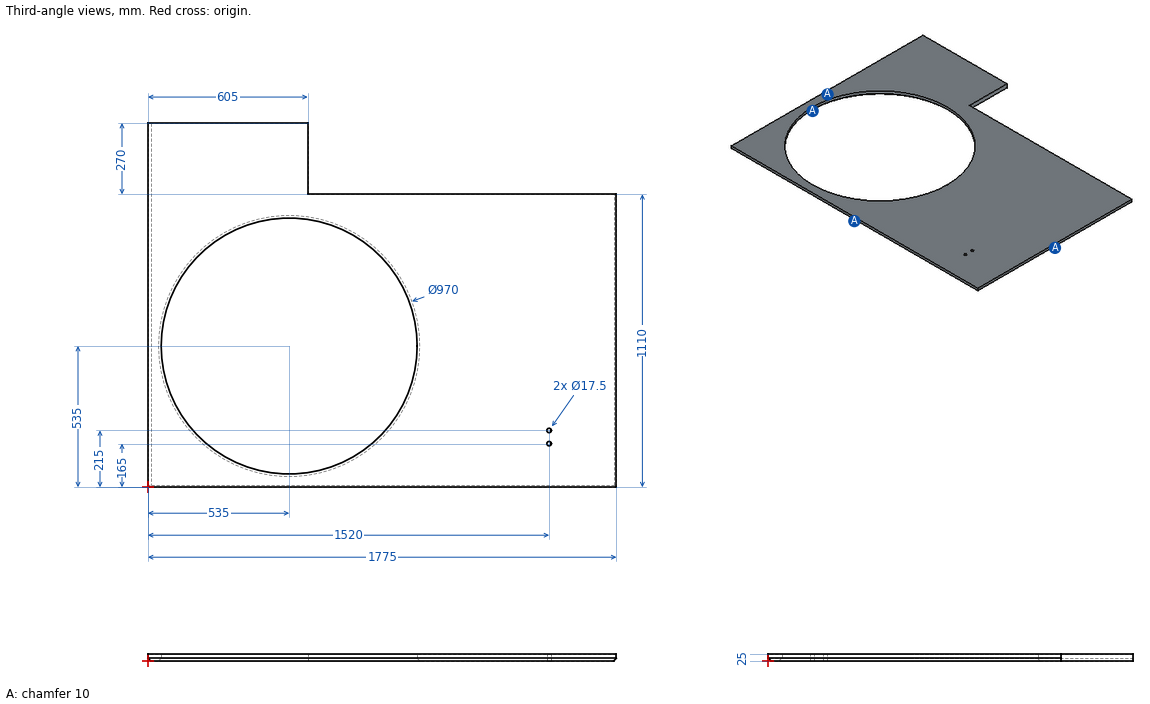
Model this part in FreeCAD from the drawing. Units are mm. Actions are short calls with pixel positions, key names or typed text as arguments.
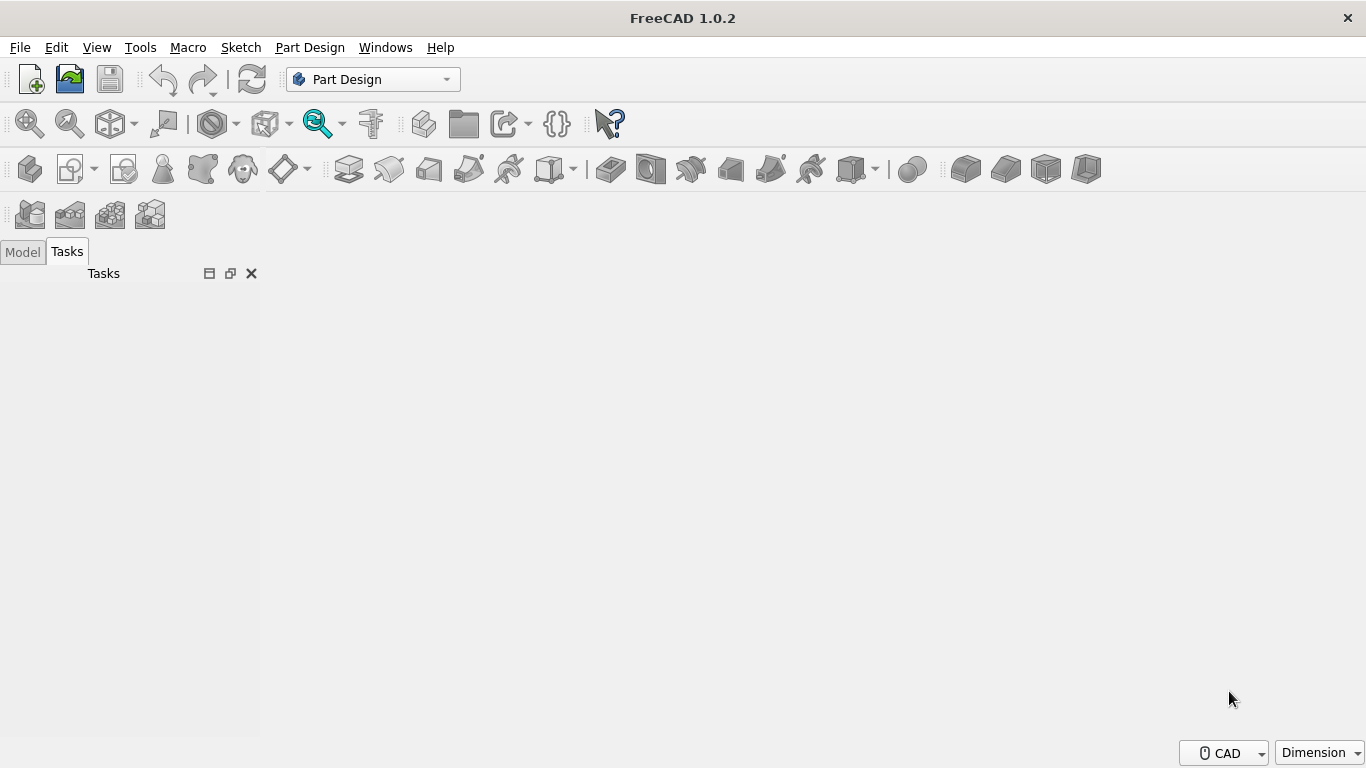
click(30, 80)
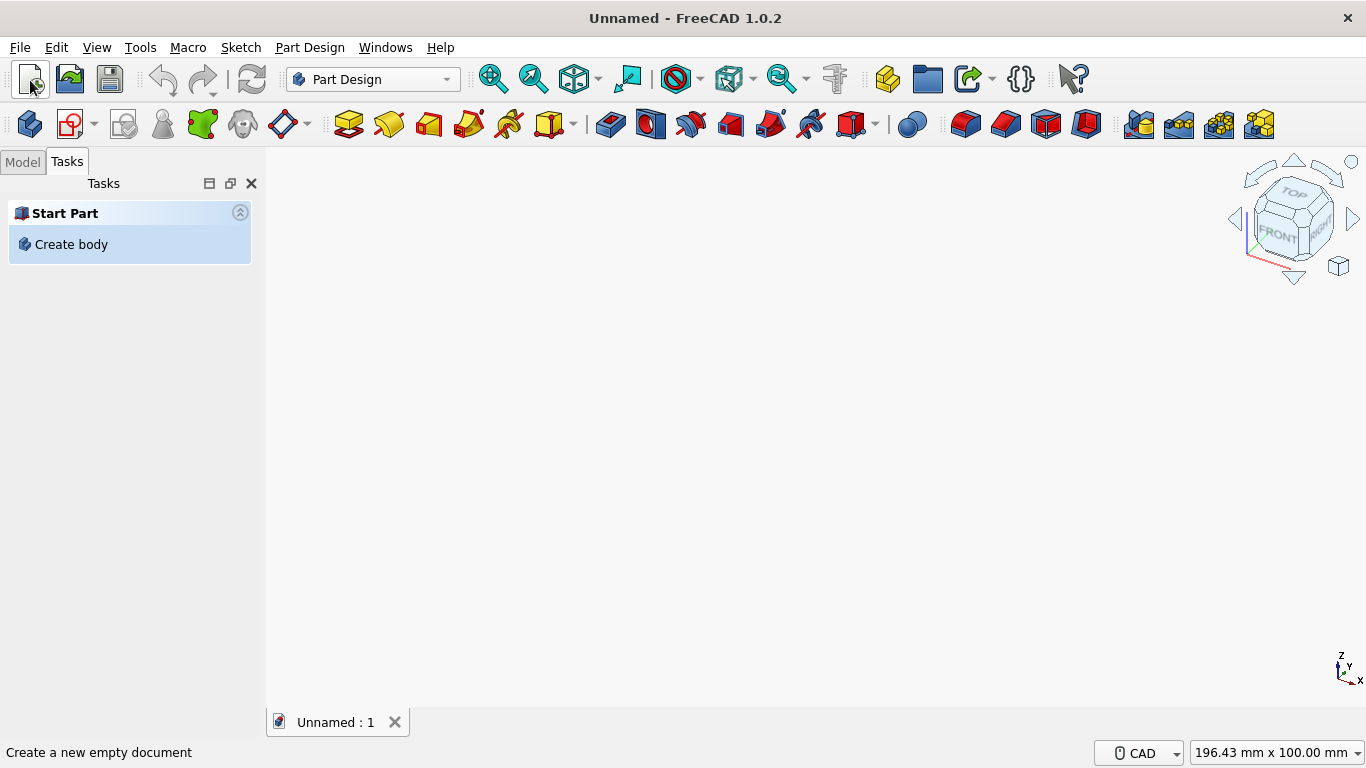
click(70, 124)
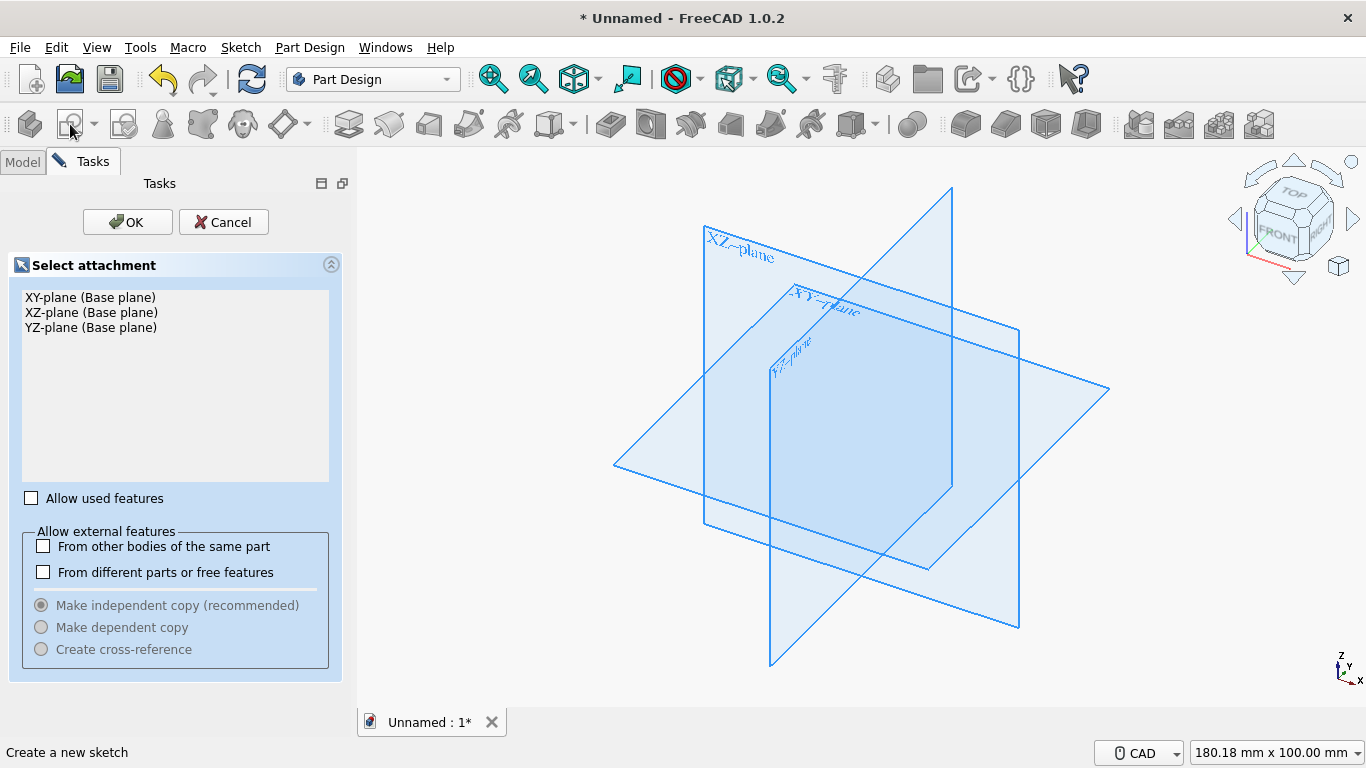
click(82, 298)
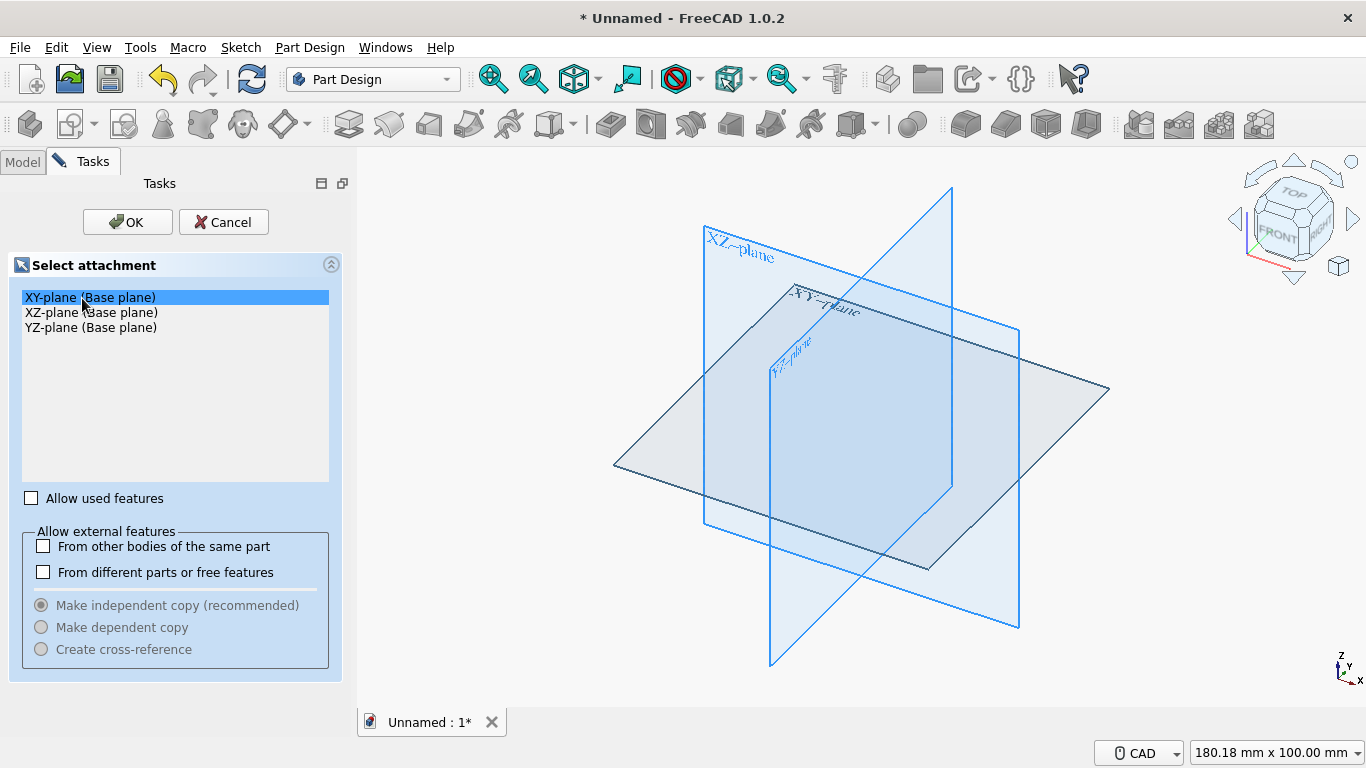
click(128, 222)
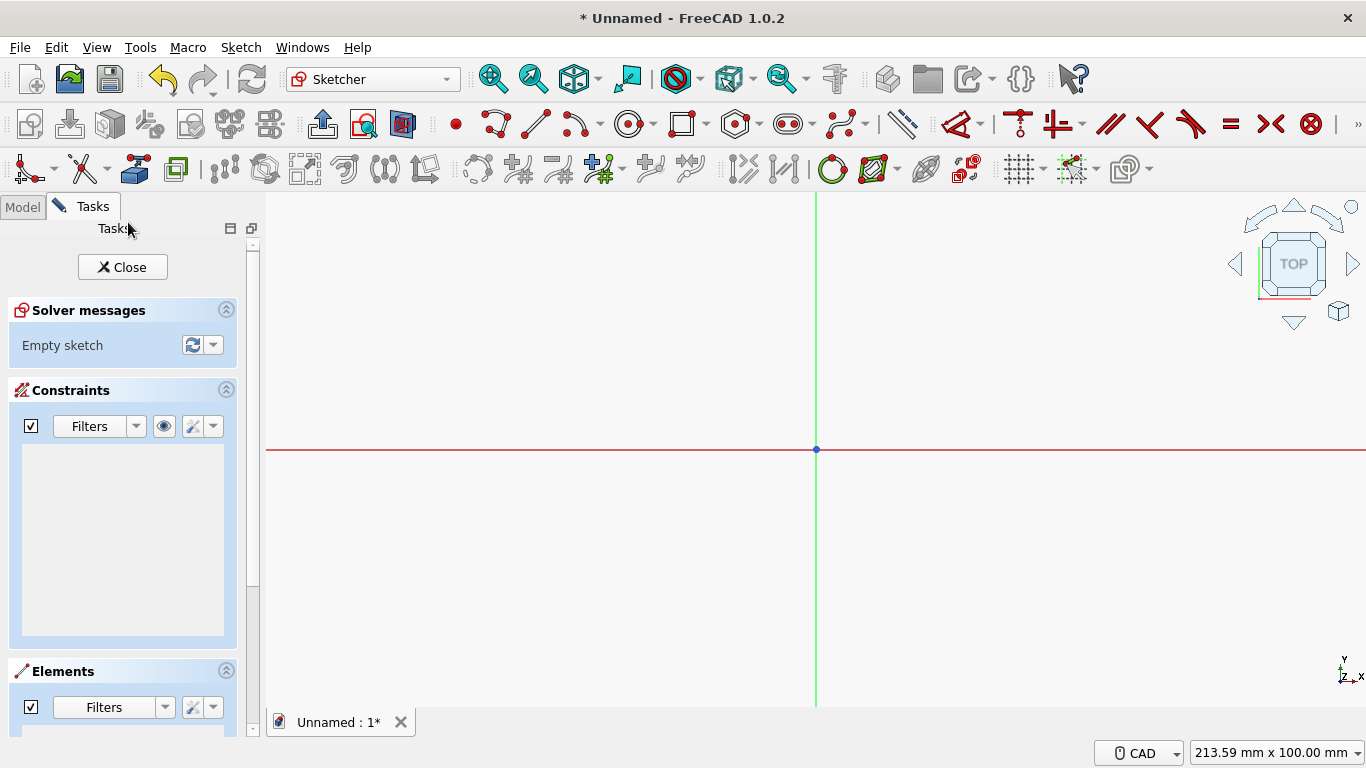
scroll(504, 636, down, 15)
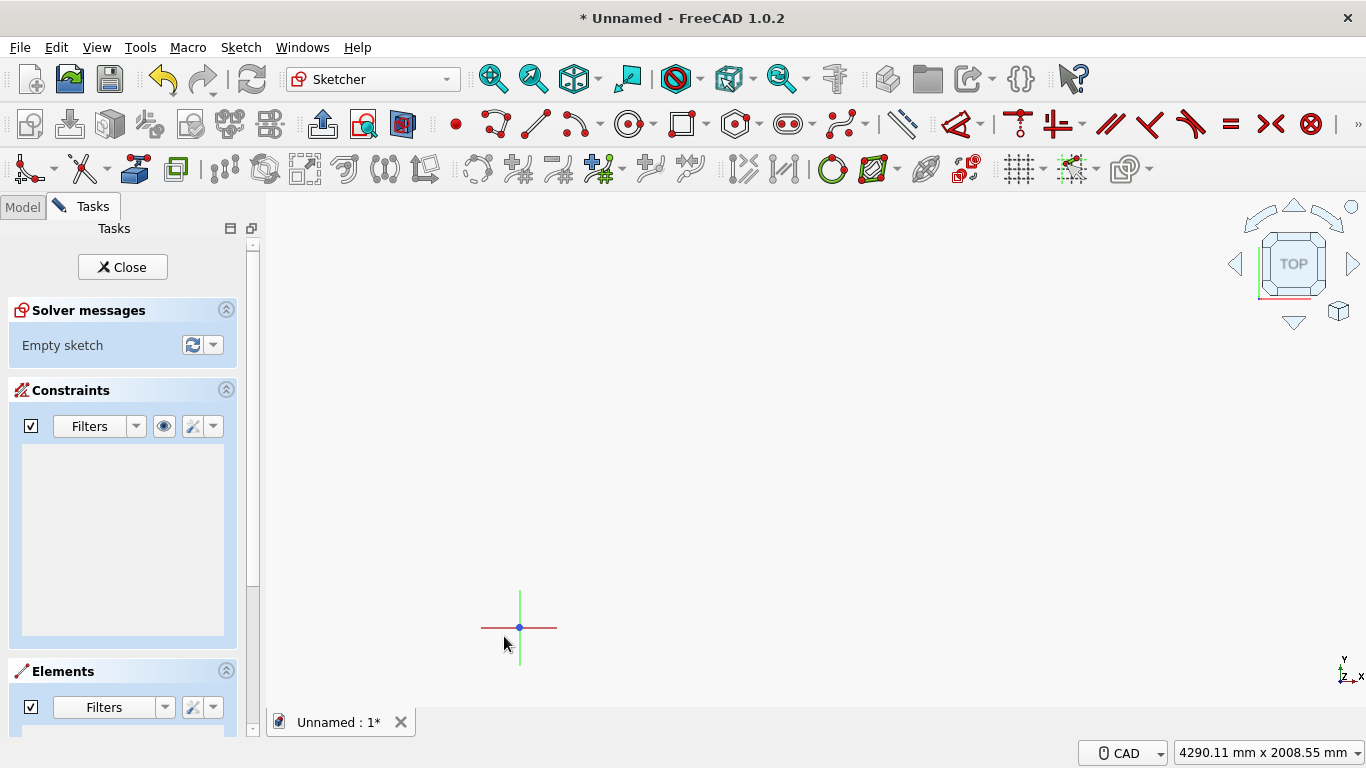
click(496, 124)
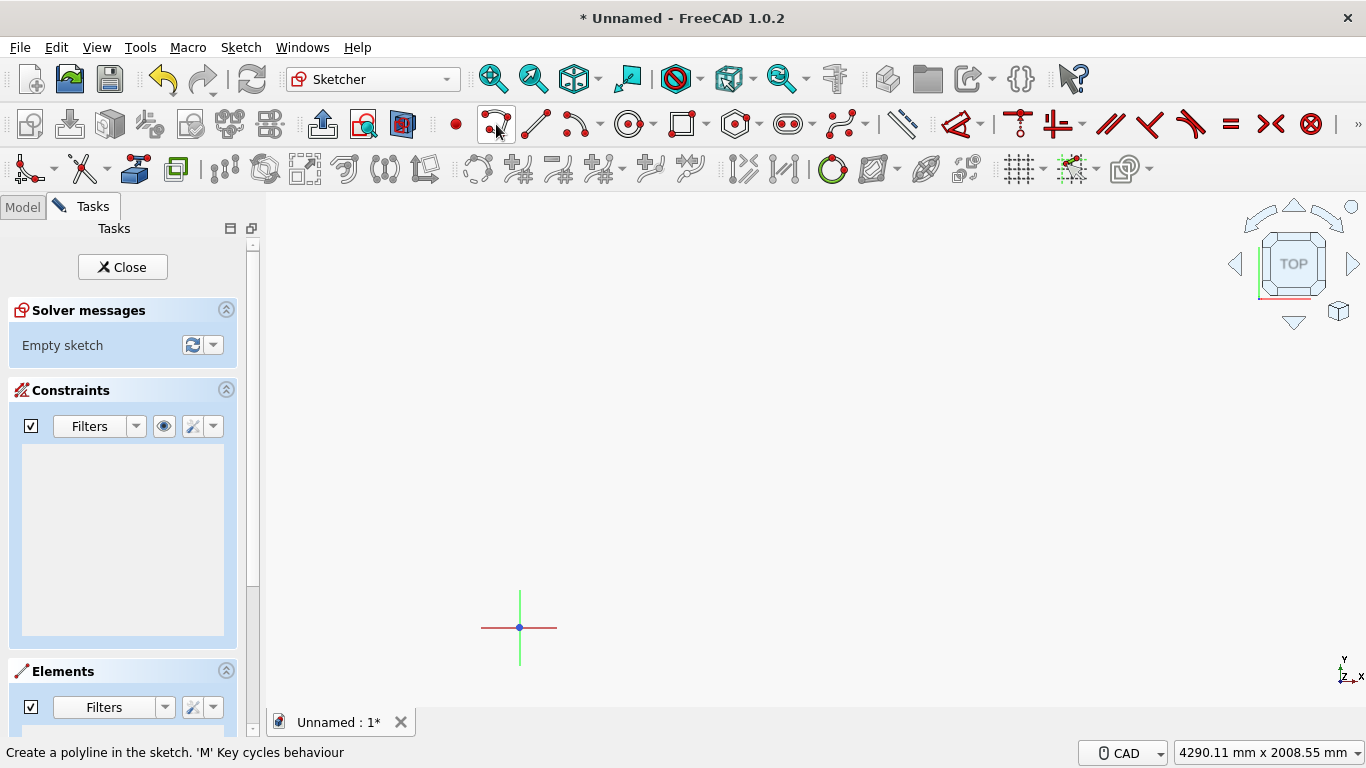
click(520, 628)
click(975, 619)
click(975, 343)
click(675, 343)
click(675, 274)
click(529, 274)
click(520, 628)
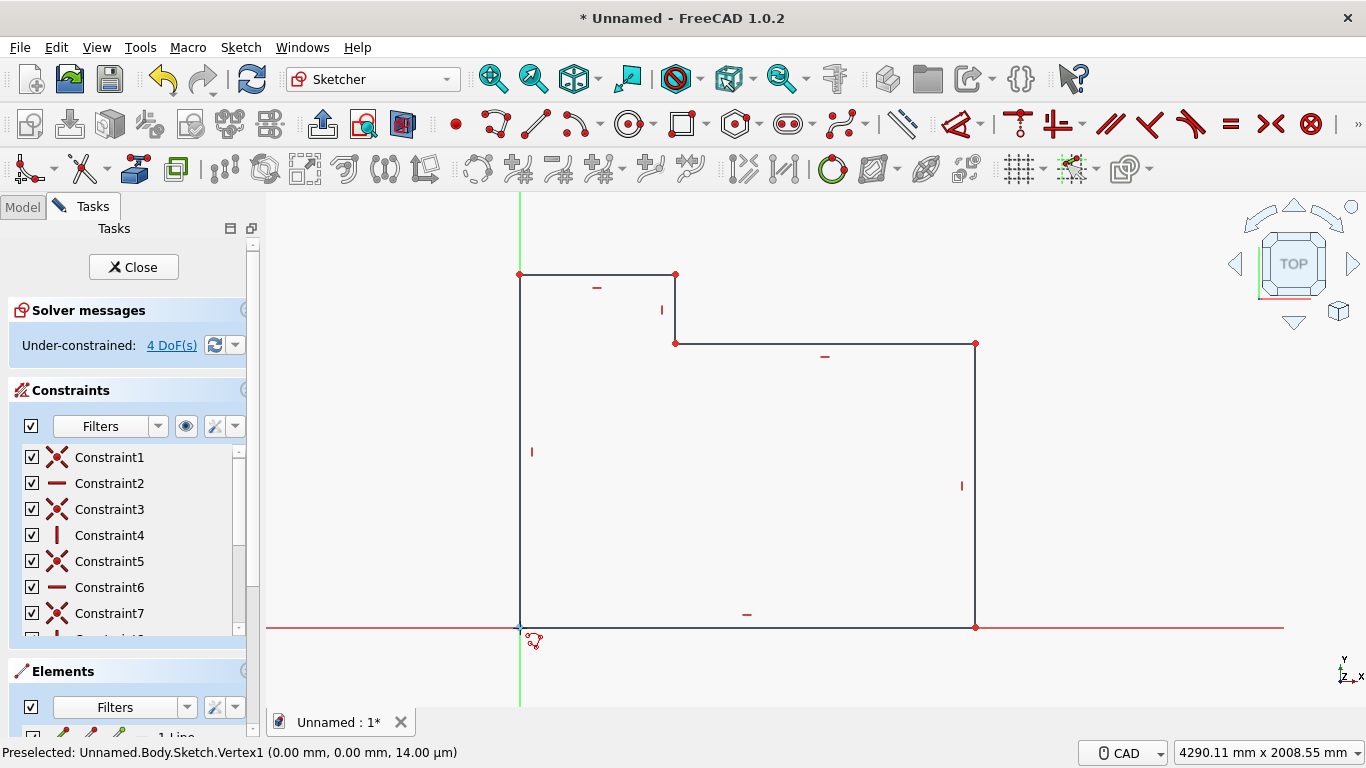
click(630, 124)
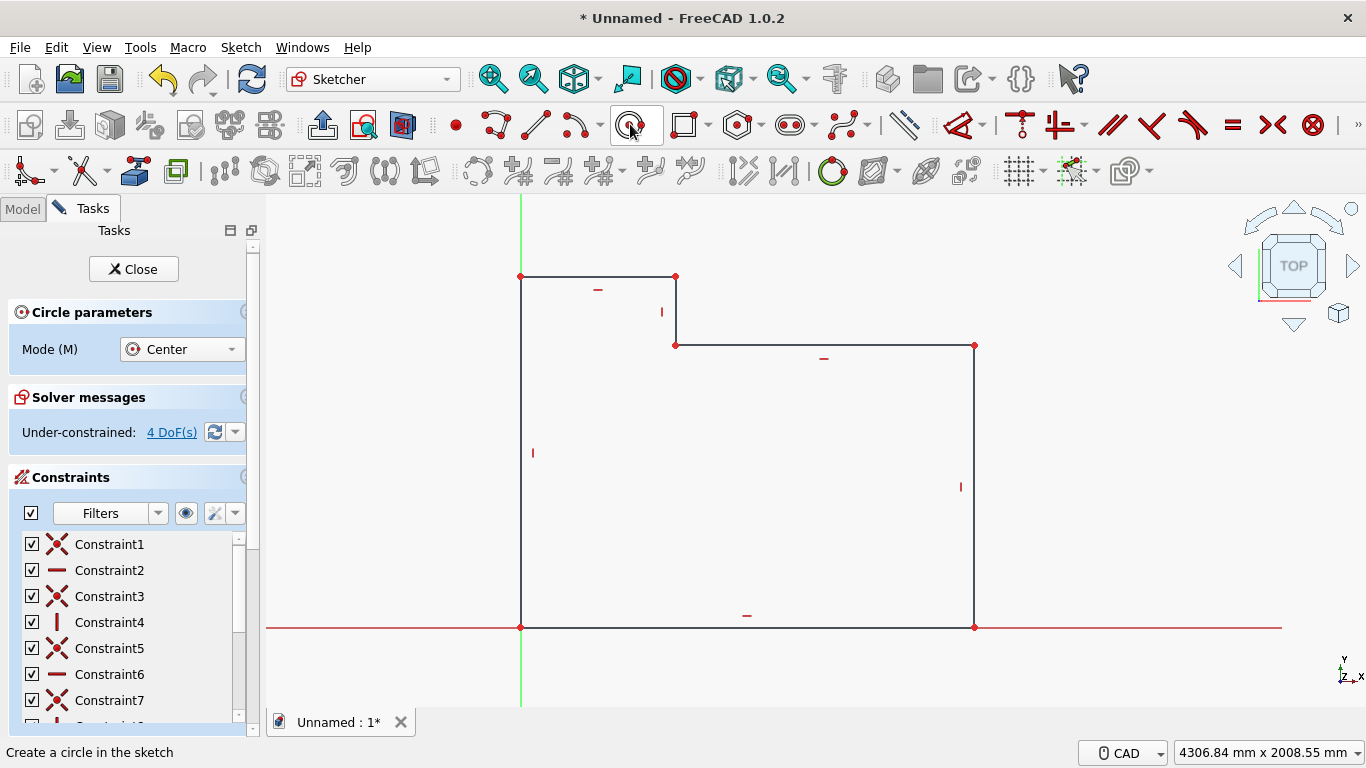
click(658, 491)
click(745, 404)
key(Escape)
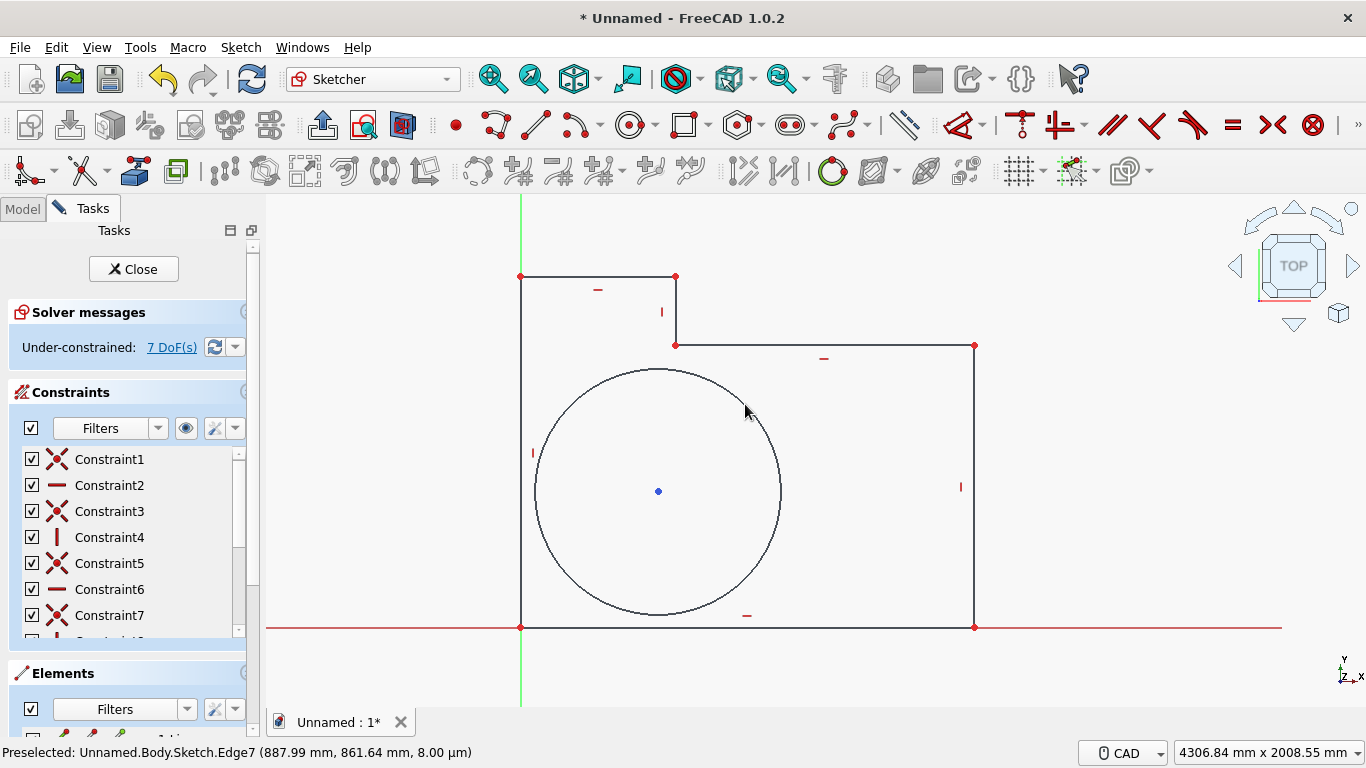
click(745, 405)